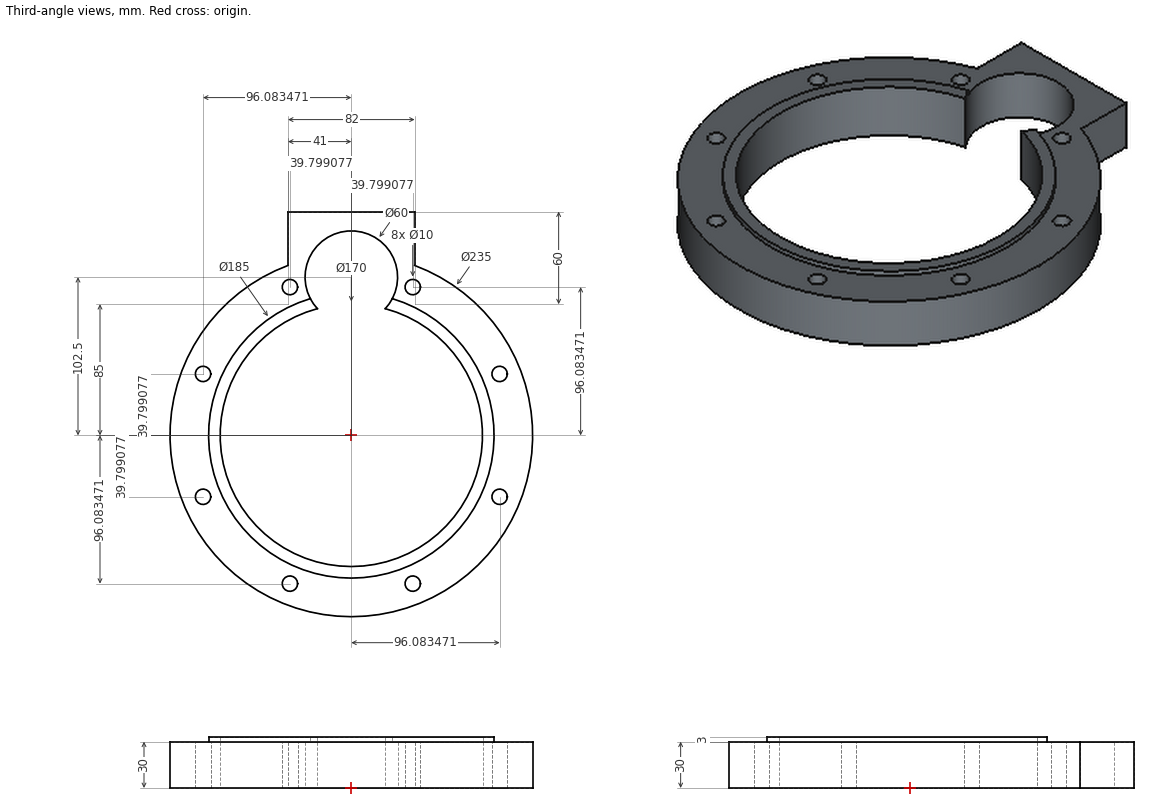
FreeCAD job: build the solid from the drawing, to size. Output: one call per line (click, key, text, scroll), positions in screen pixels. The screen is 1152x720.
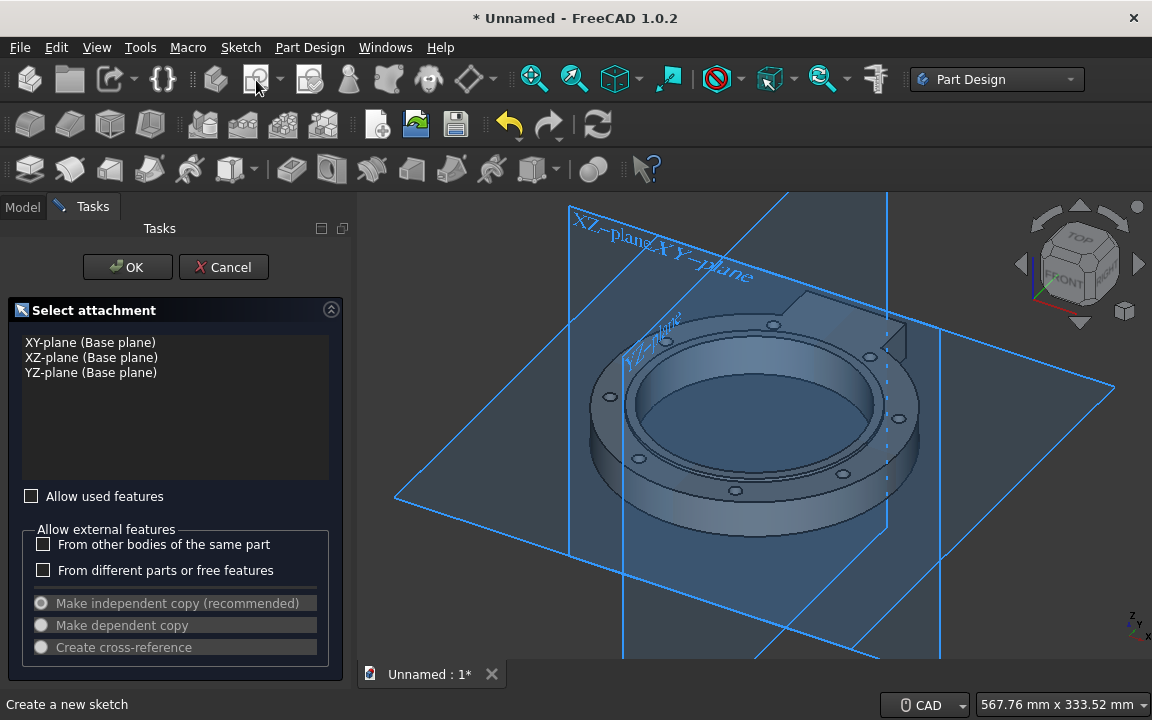
click(82, 342)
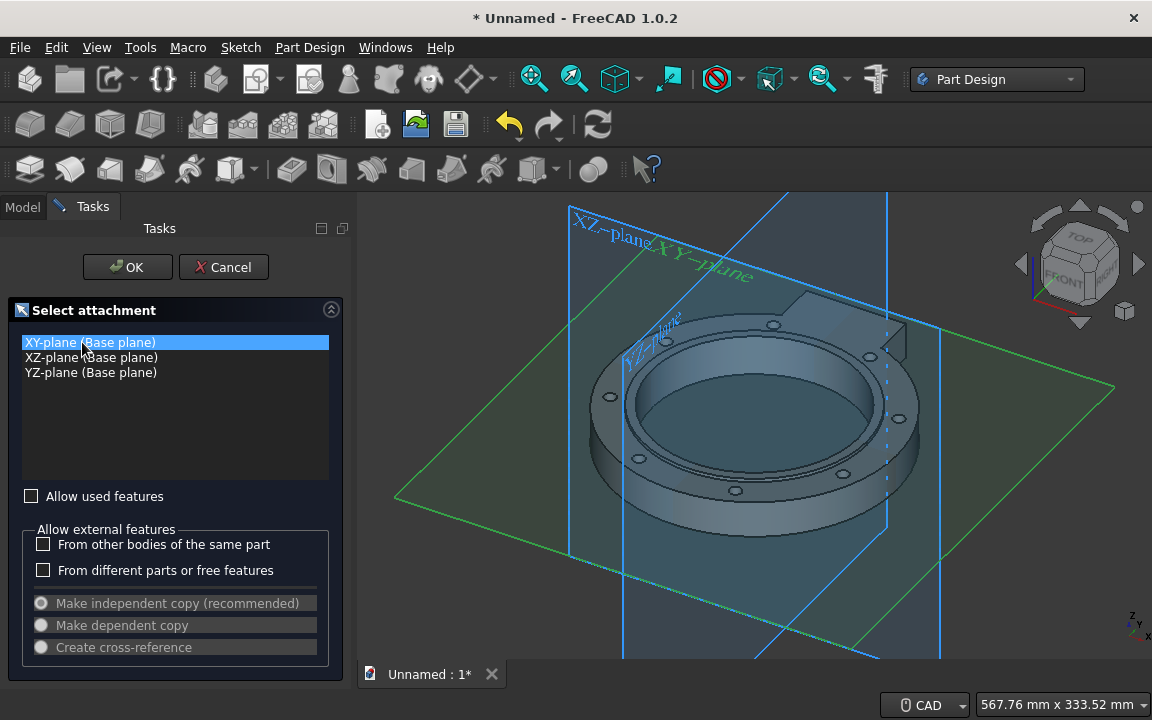
click(128, 267)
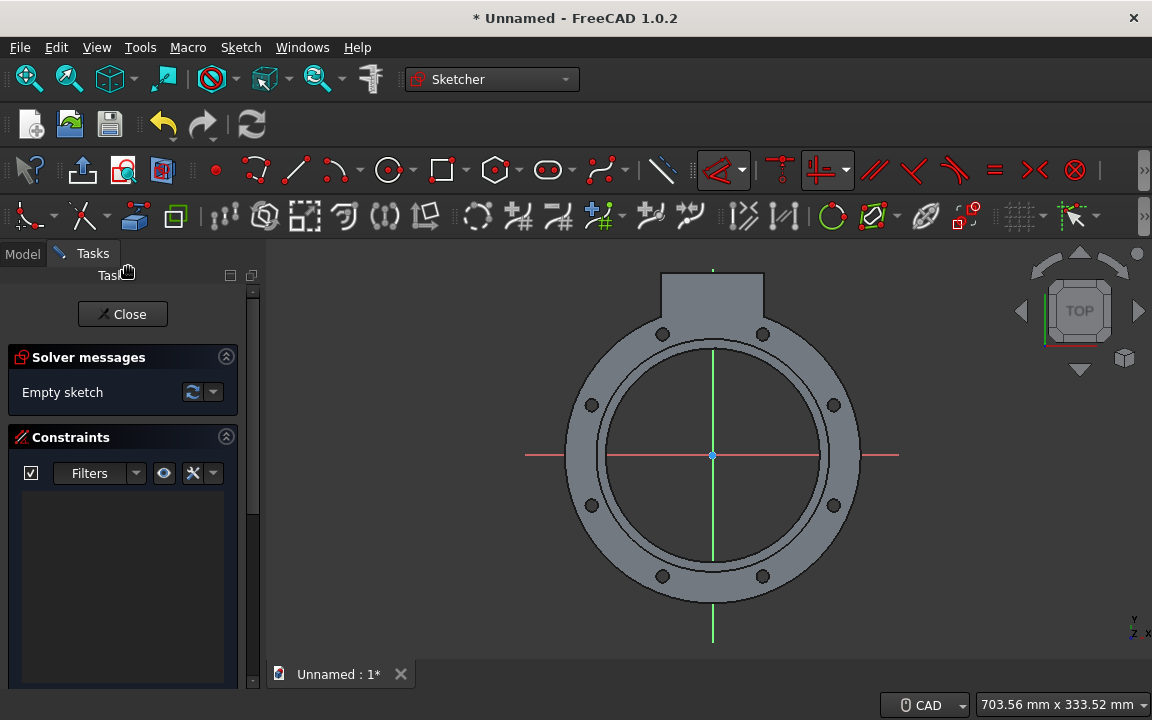
click(164, 170)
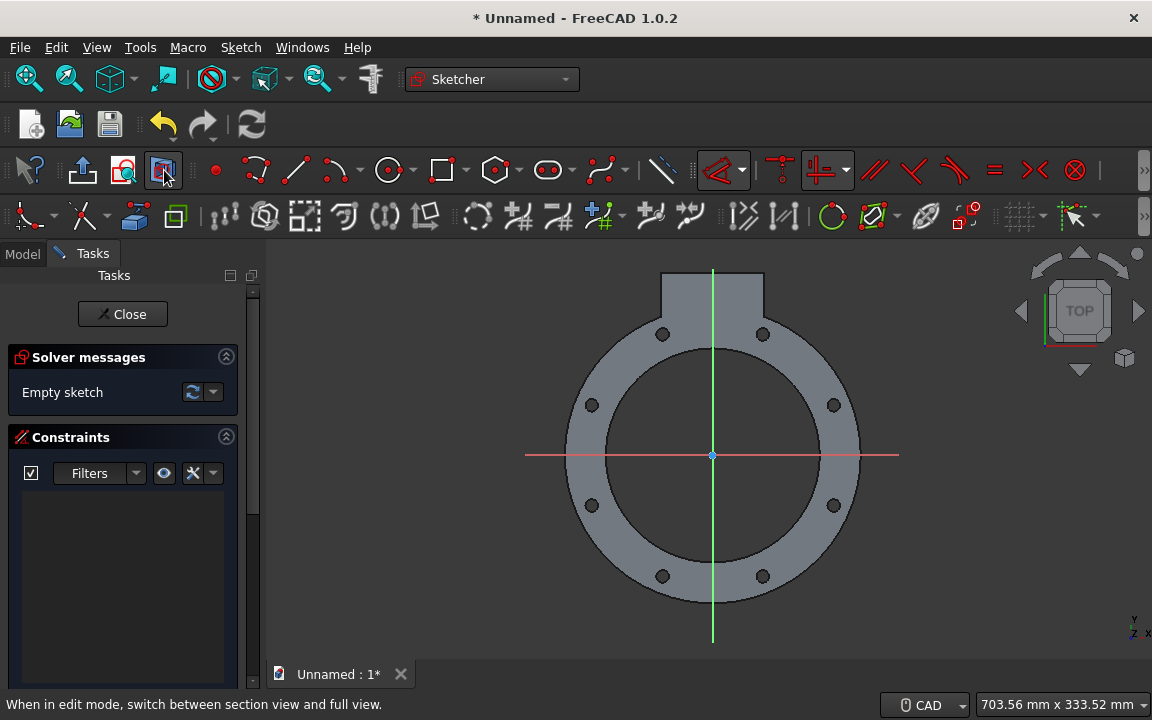
scroll(860, 267, up, 2)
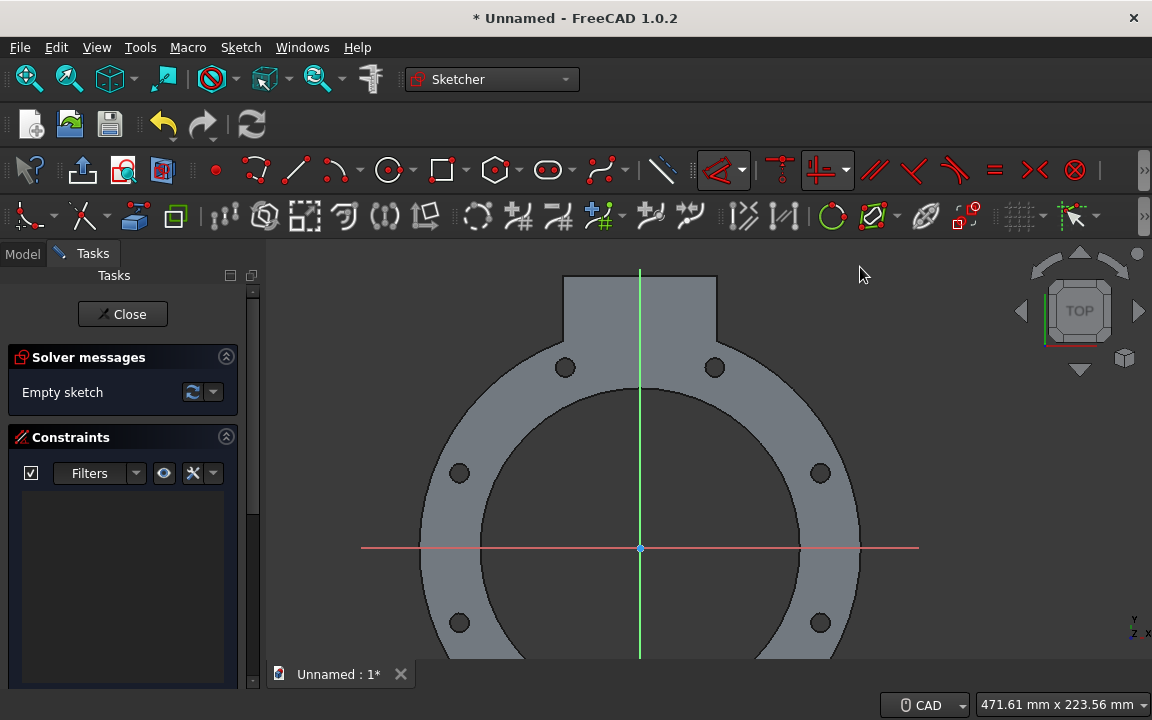
key(g)
key(c)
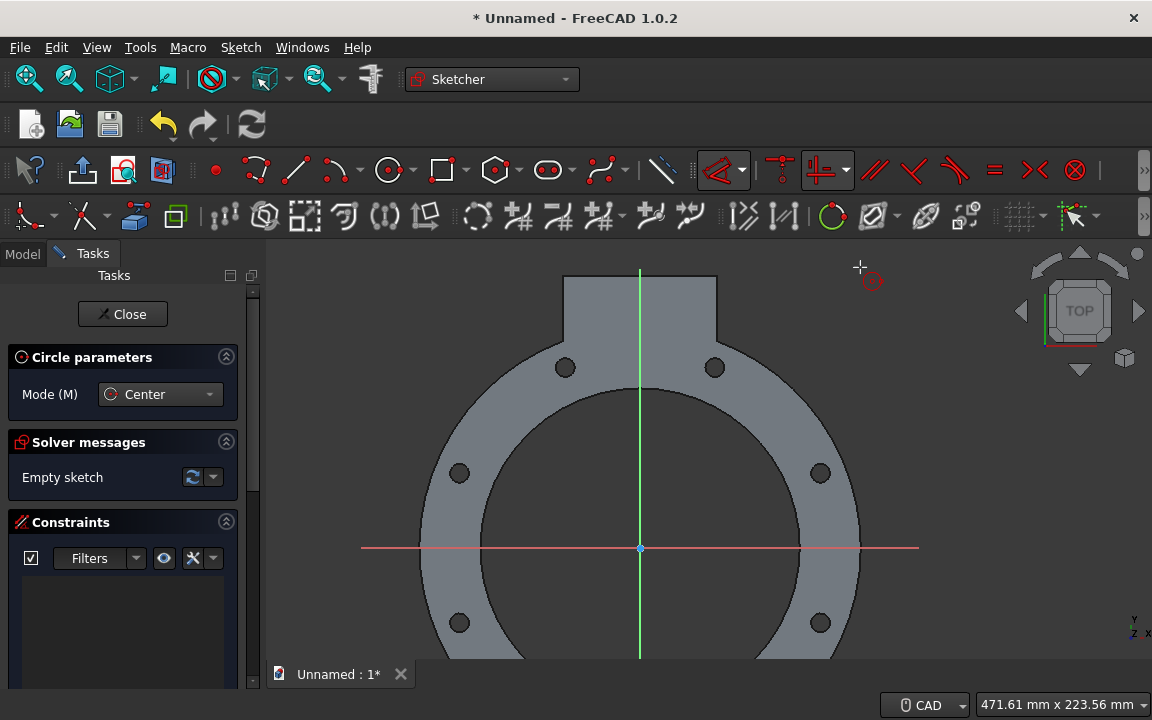
click(640, 356)
move(680, 316)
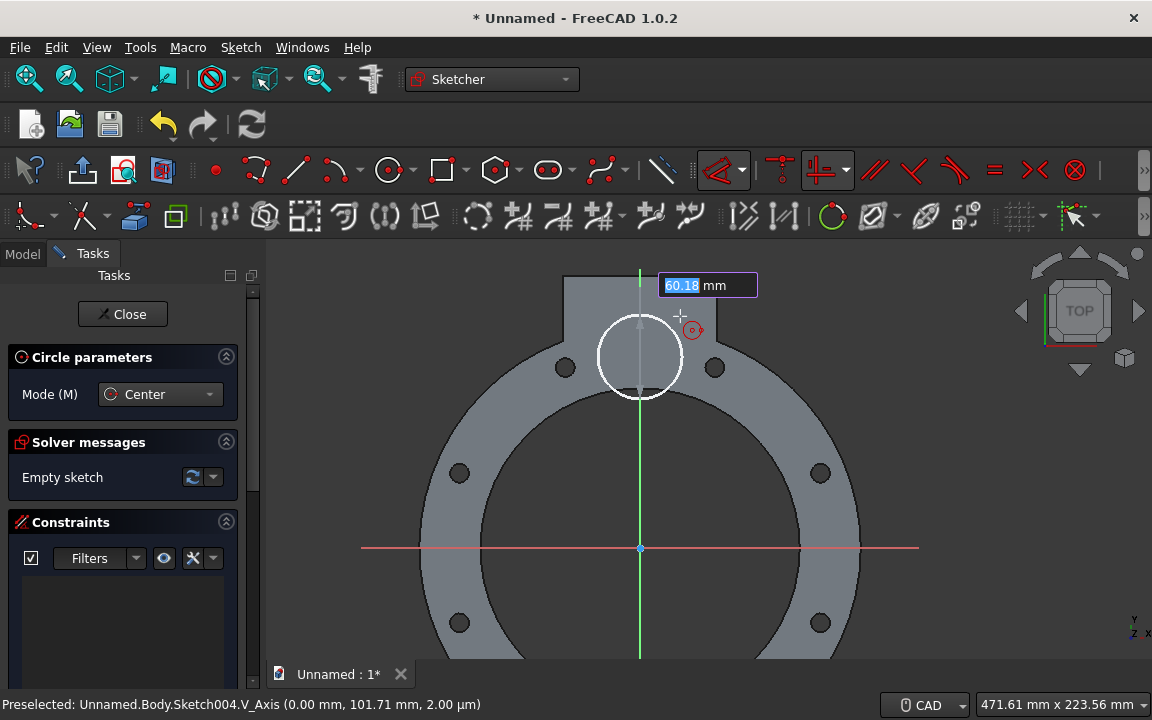
text(60)
key(Return)
key(Escape)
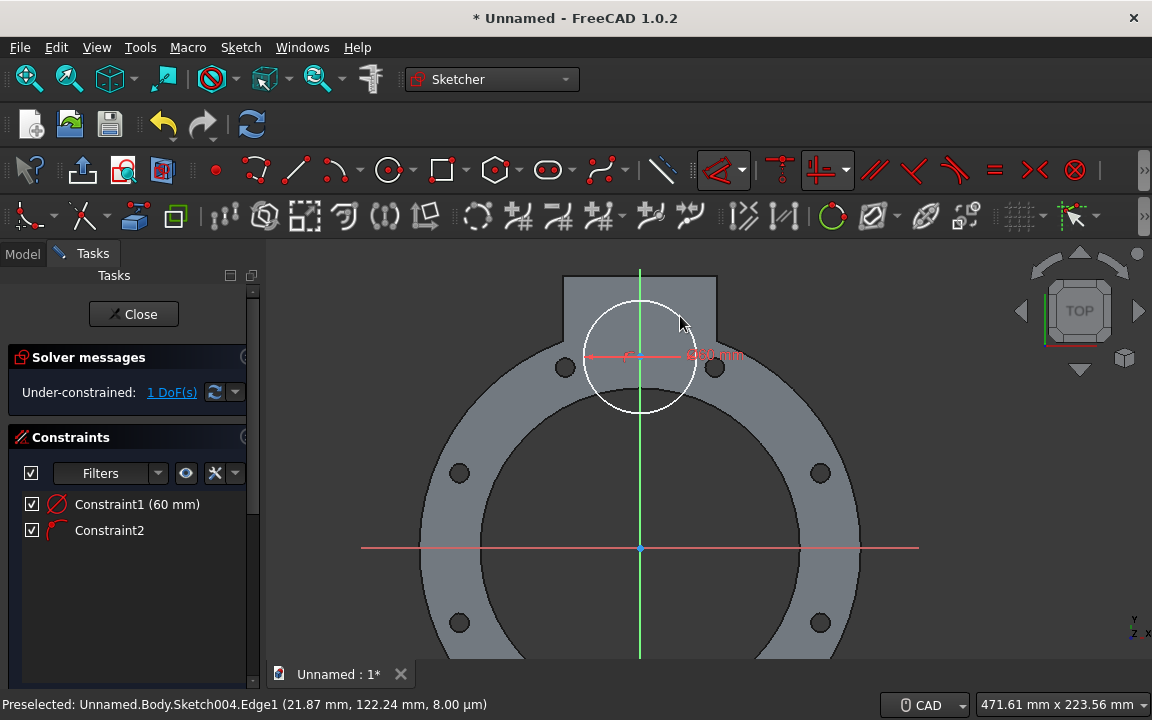
click(640, 357)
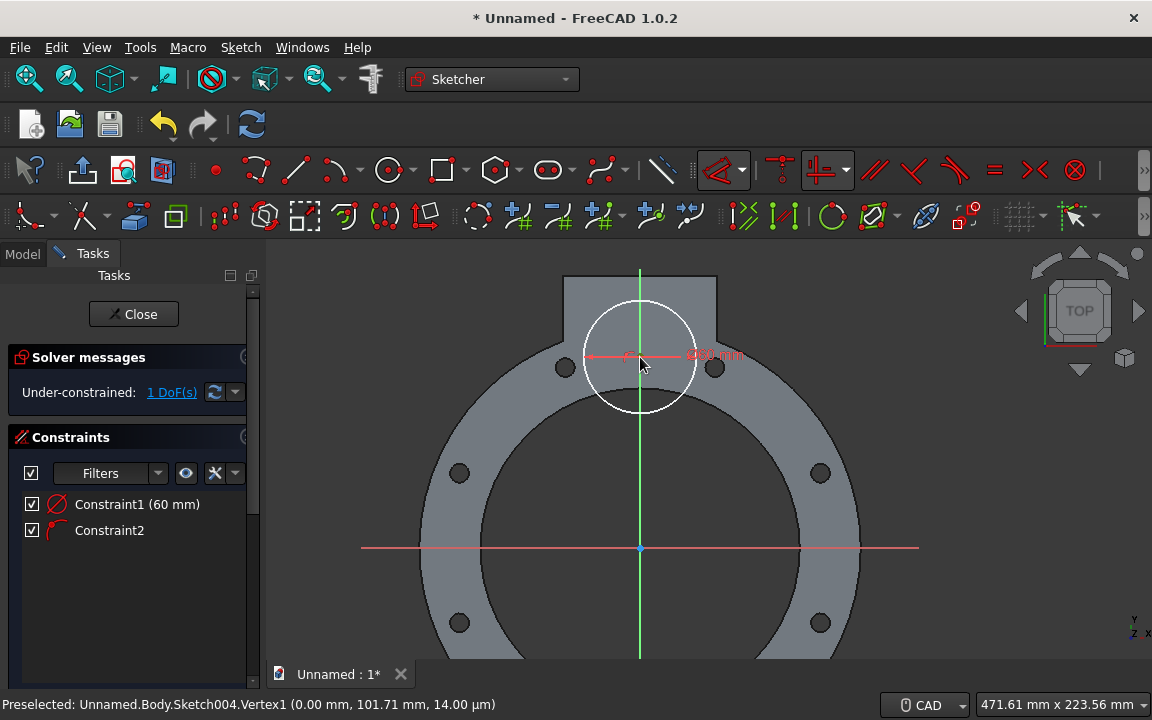
click(744, 170)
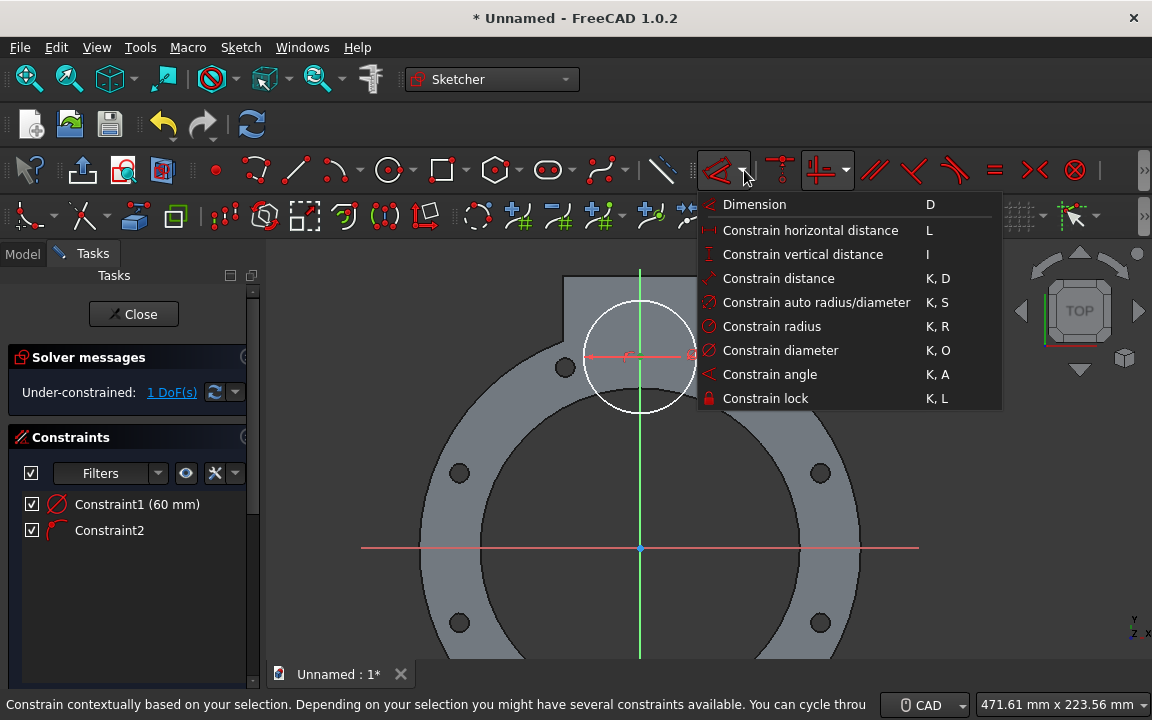
click(850, 254)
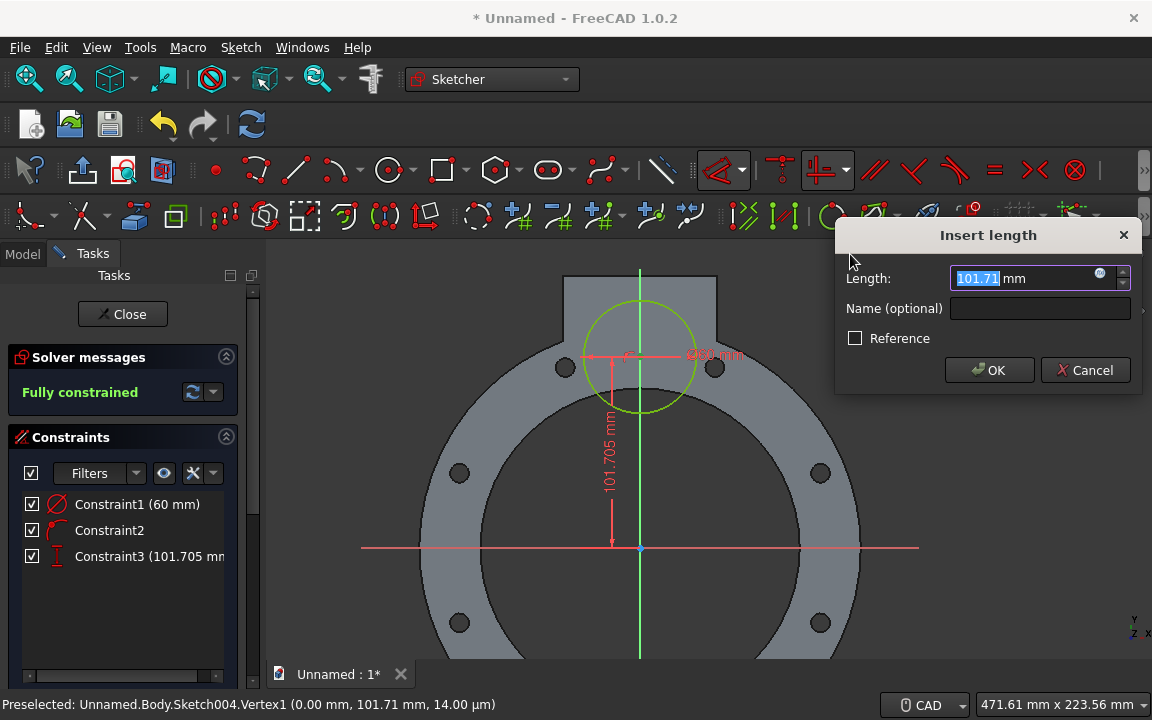
text(102.5)
key(Return)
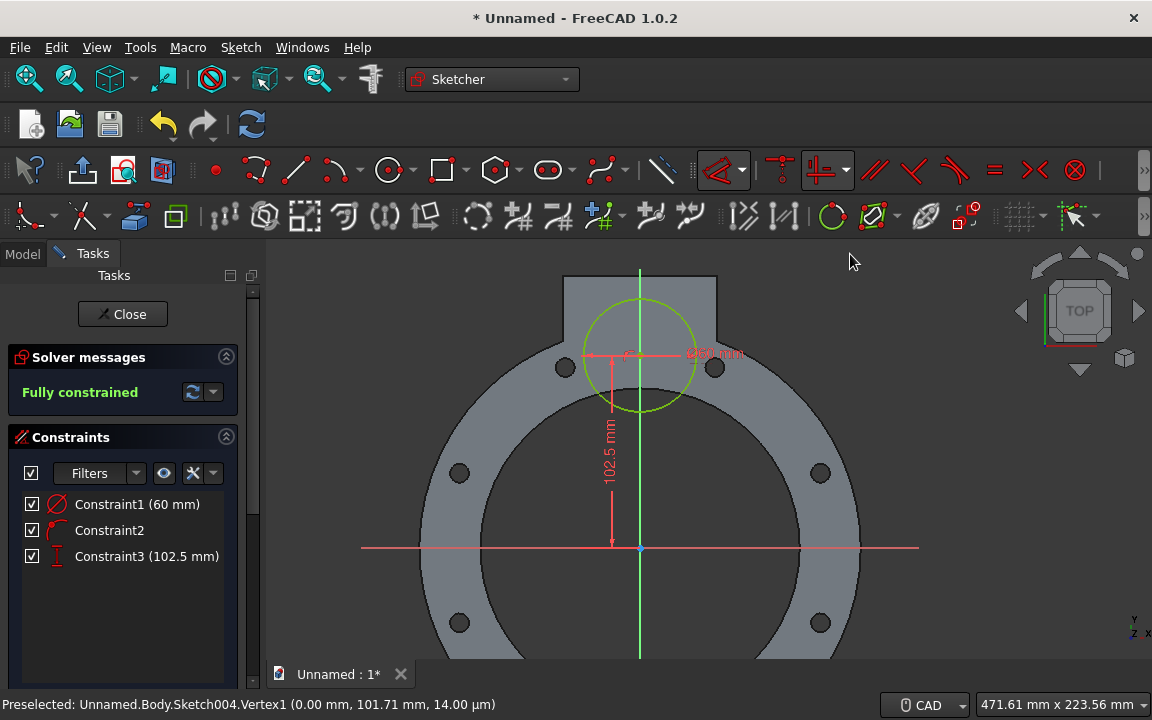
click(123, 314)